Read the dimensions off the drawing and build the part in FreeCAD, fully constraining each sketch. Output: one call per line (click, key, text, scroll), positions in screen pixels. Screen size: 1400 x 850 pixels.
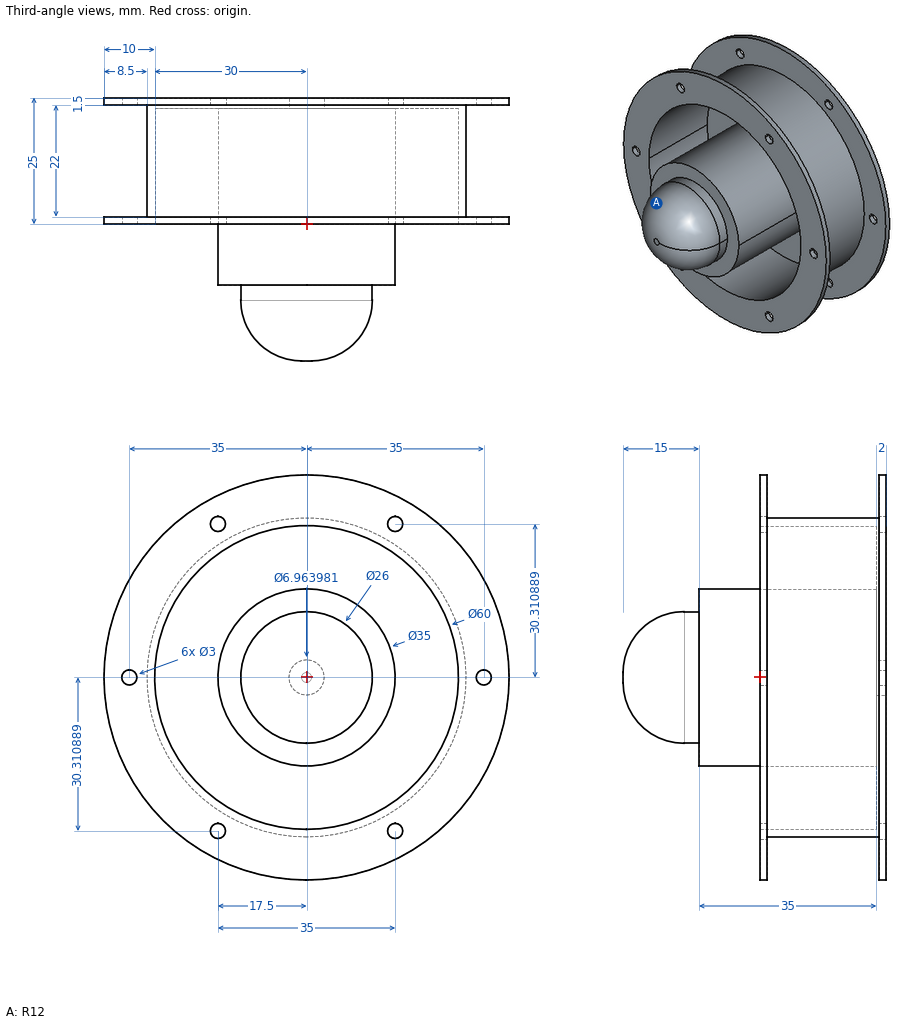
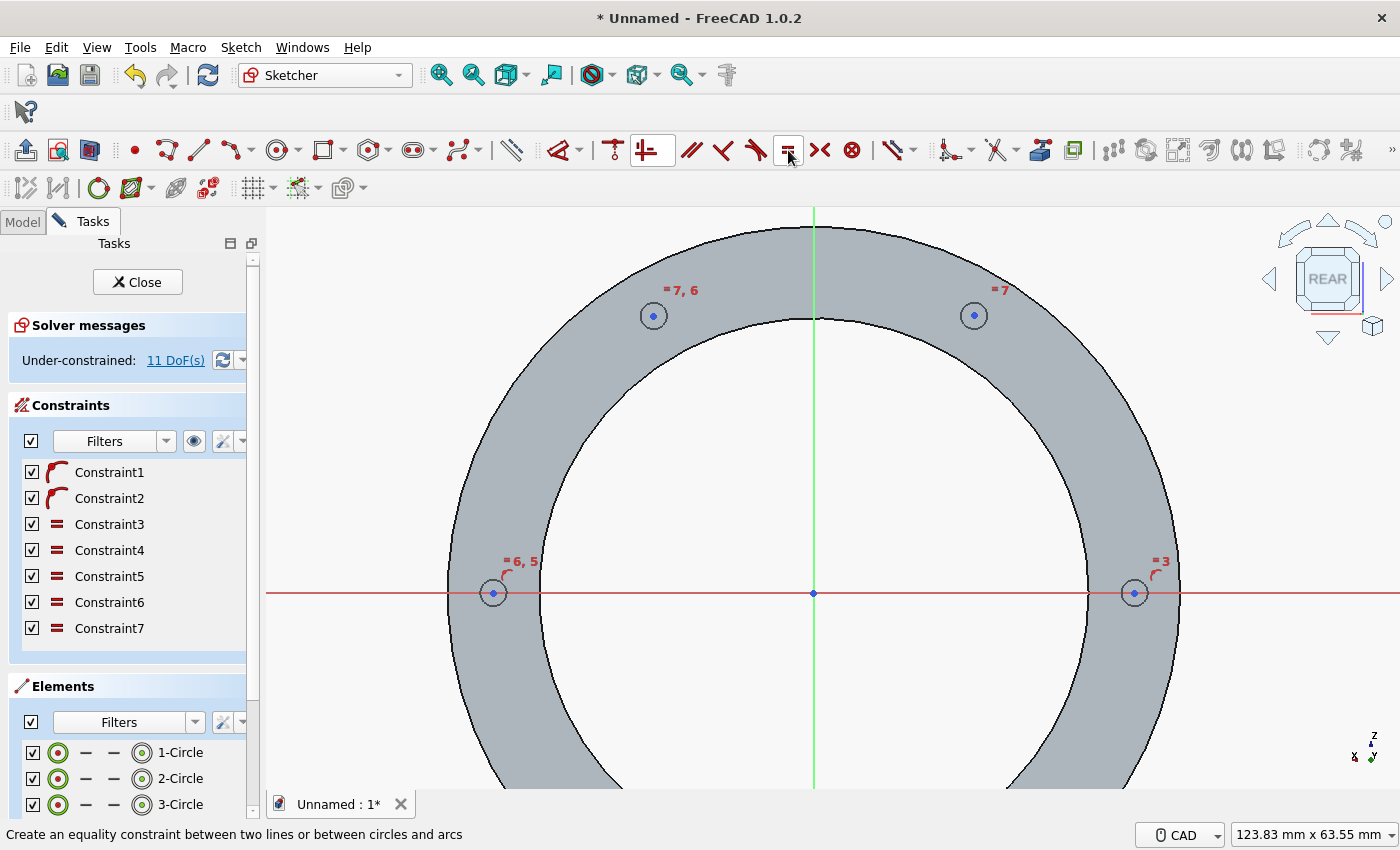
scroll(664, 305, down, 2)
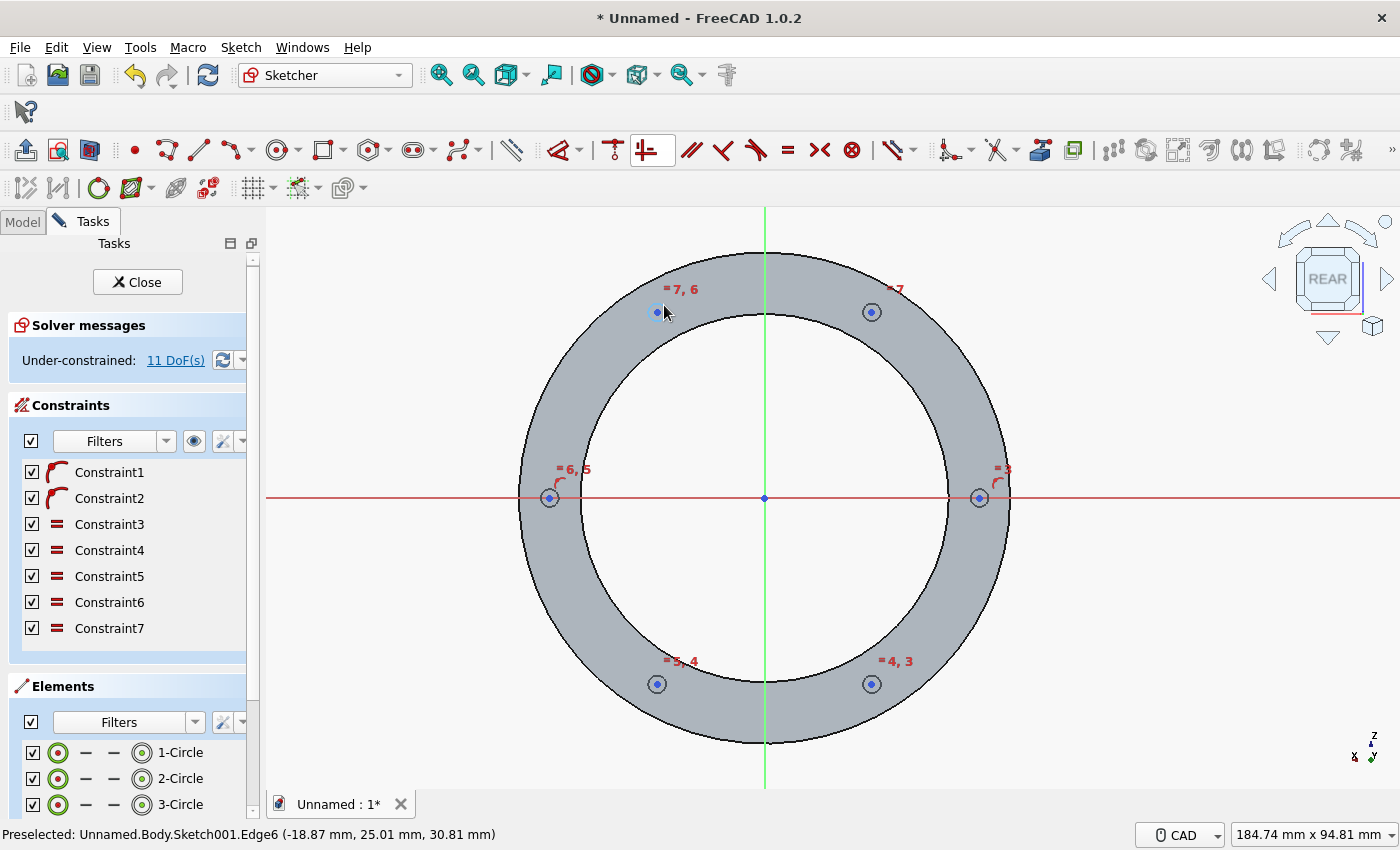
click(872, 684)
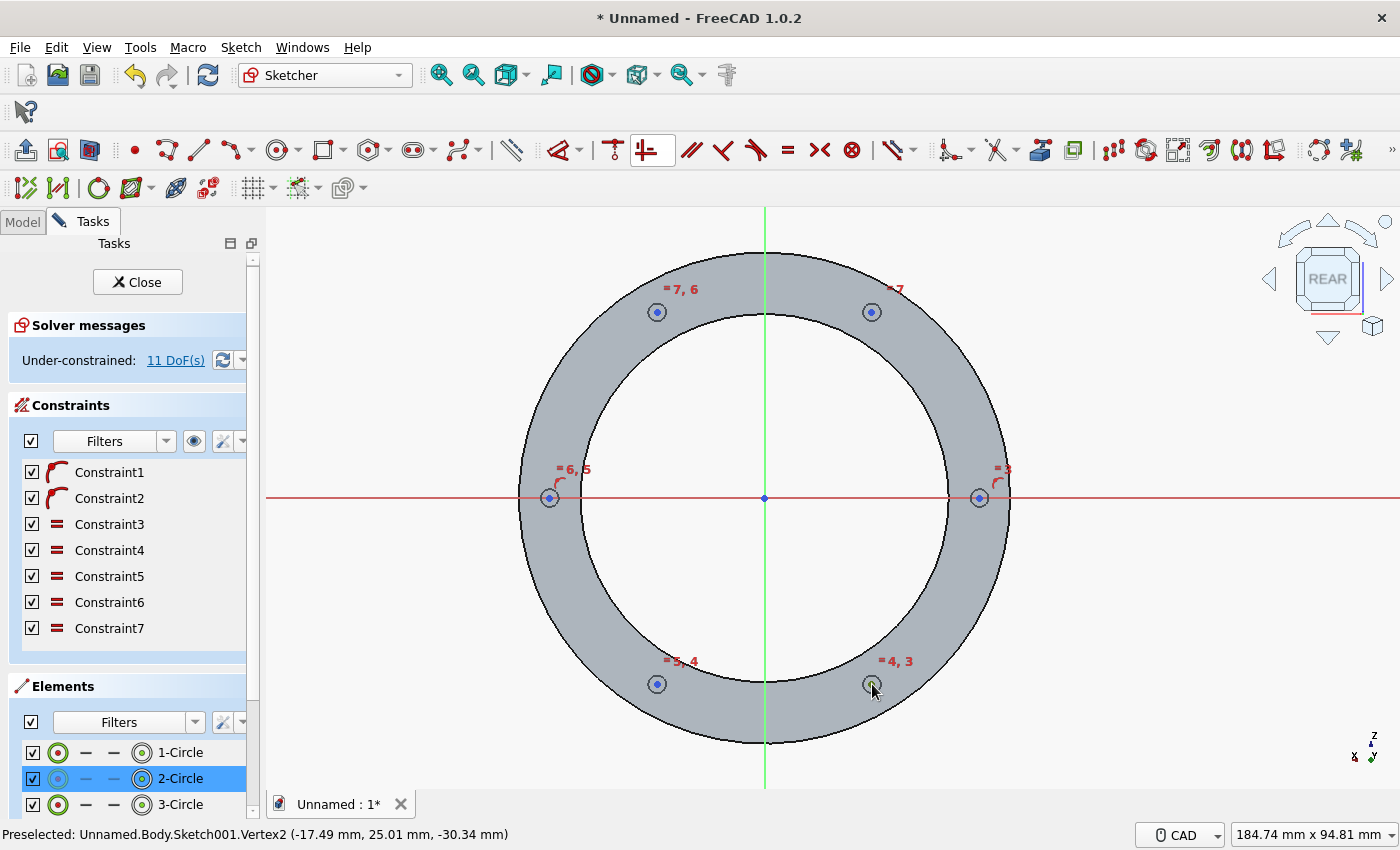
click(657, 684)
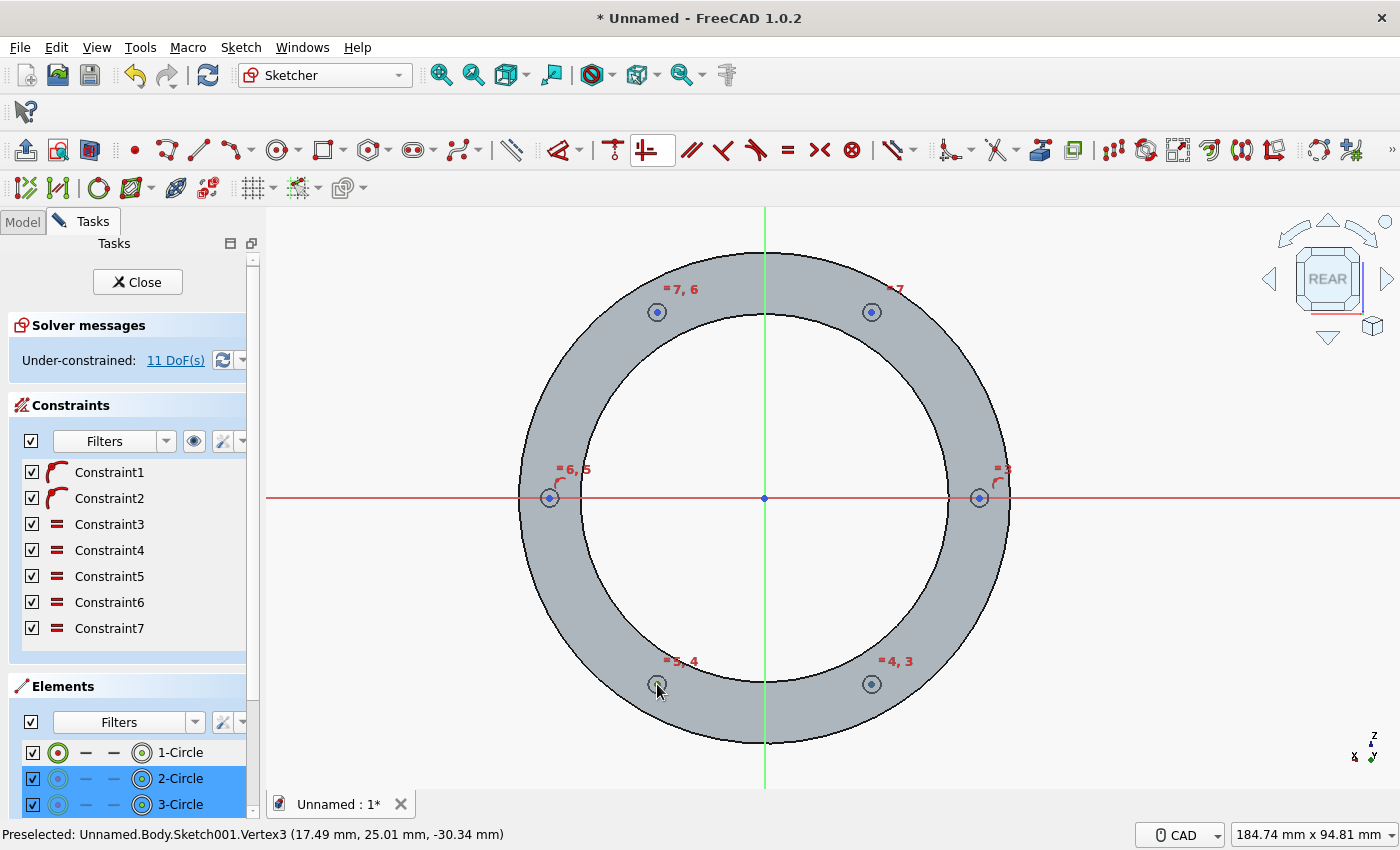
click(670, 150)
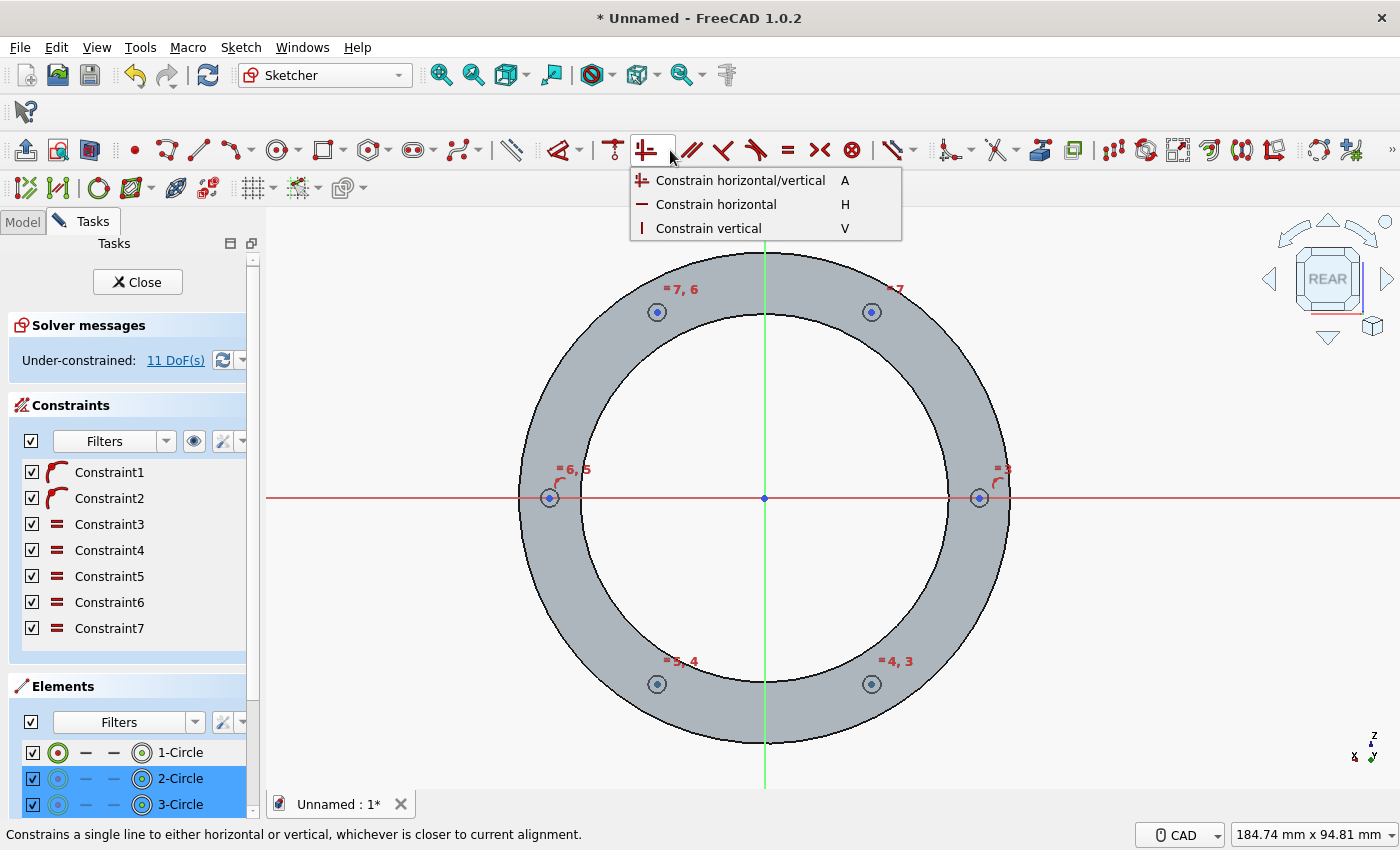
click(766, 204)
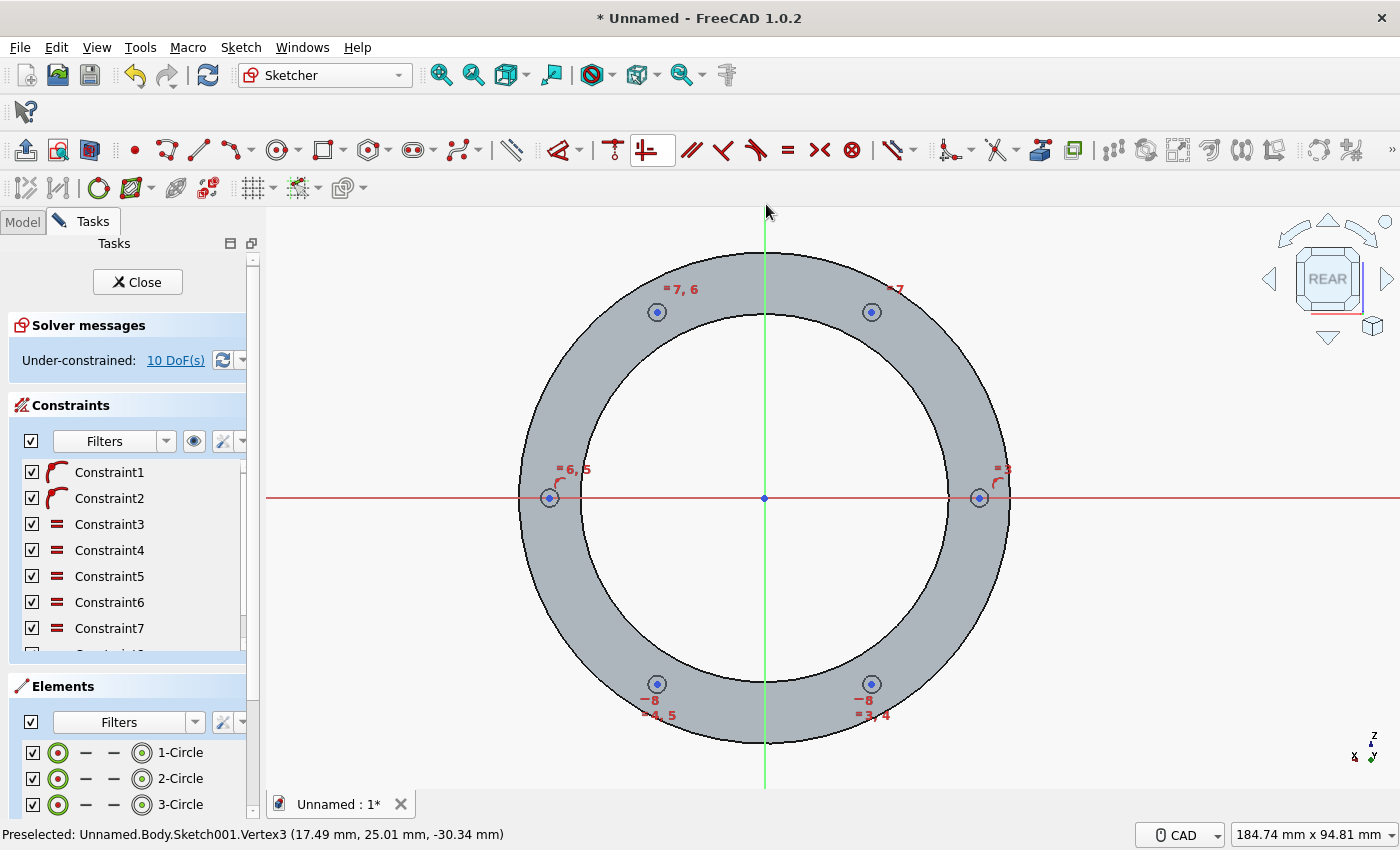
click(657, 684)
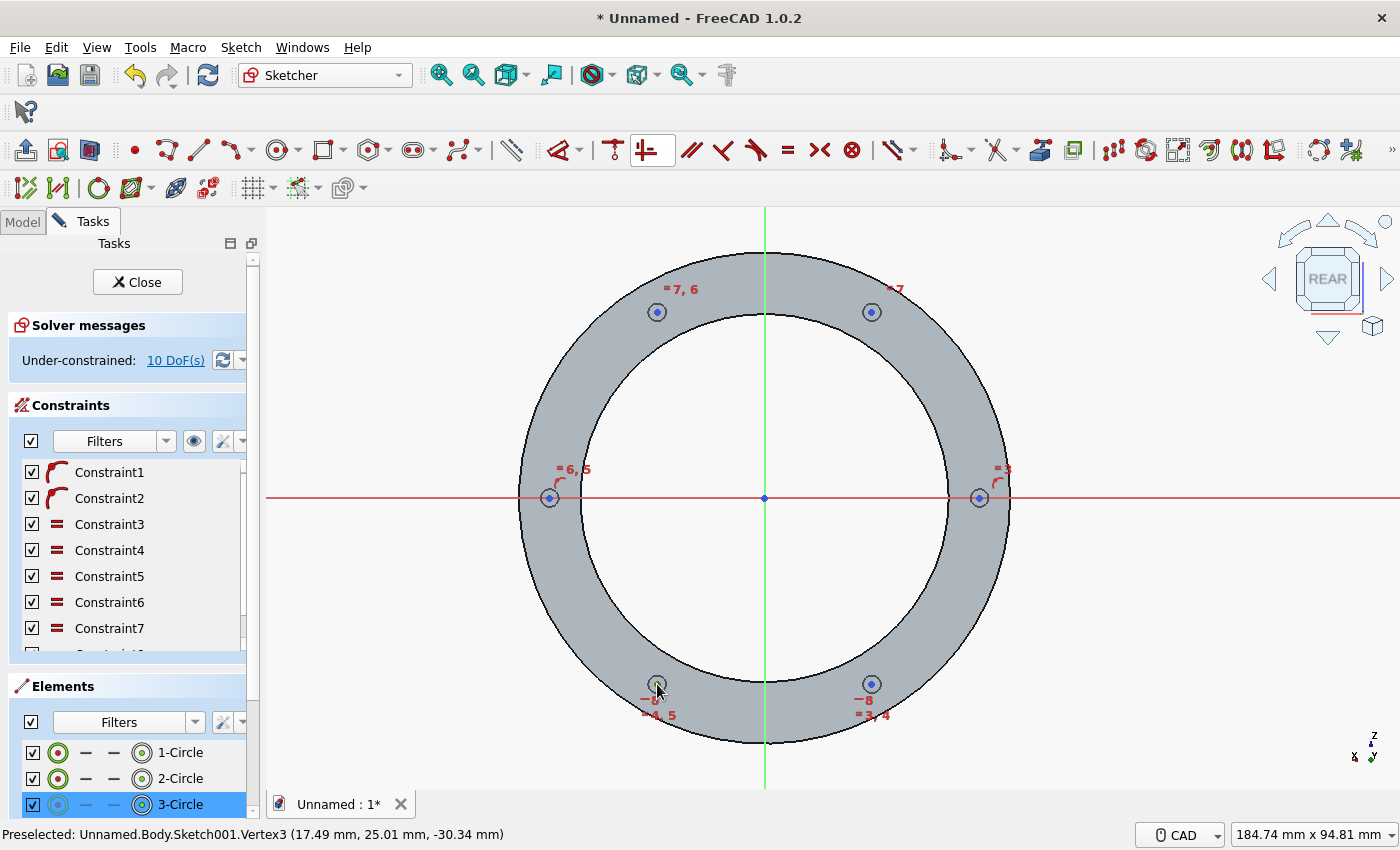
click(657, 312)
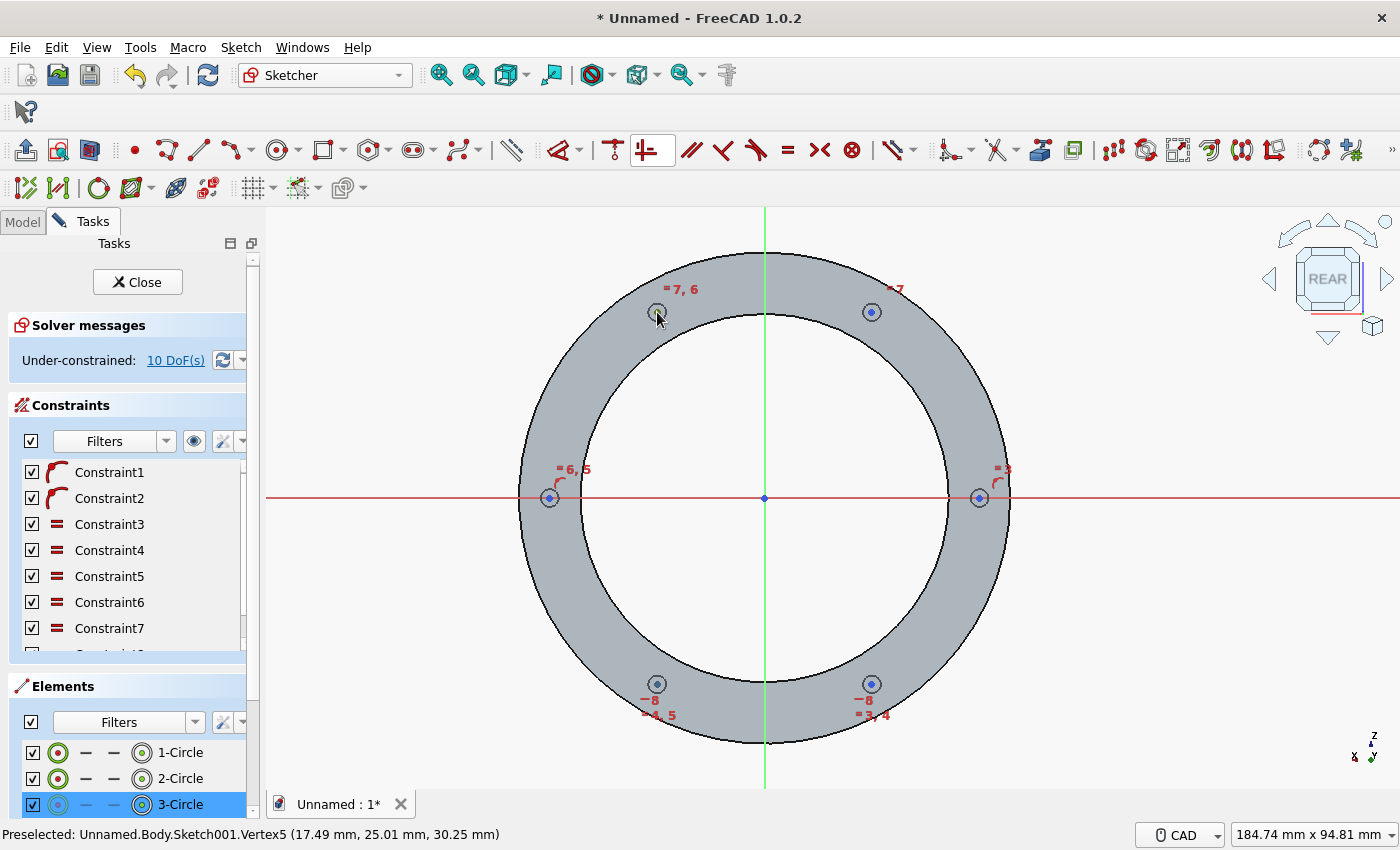
key(v)